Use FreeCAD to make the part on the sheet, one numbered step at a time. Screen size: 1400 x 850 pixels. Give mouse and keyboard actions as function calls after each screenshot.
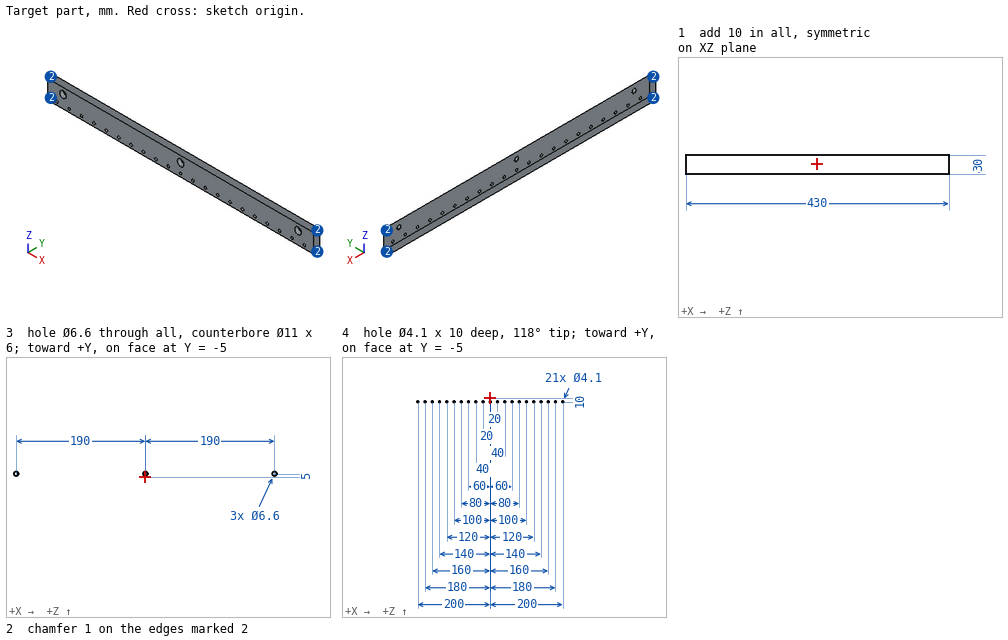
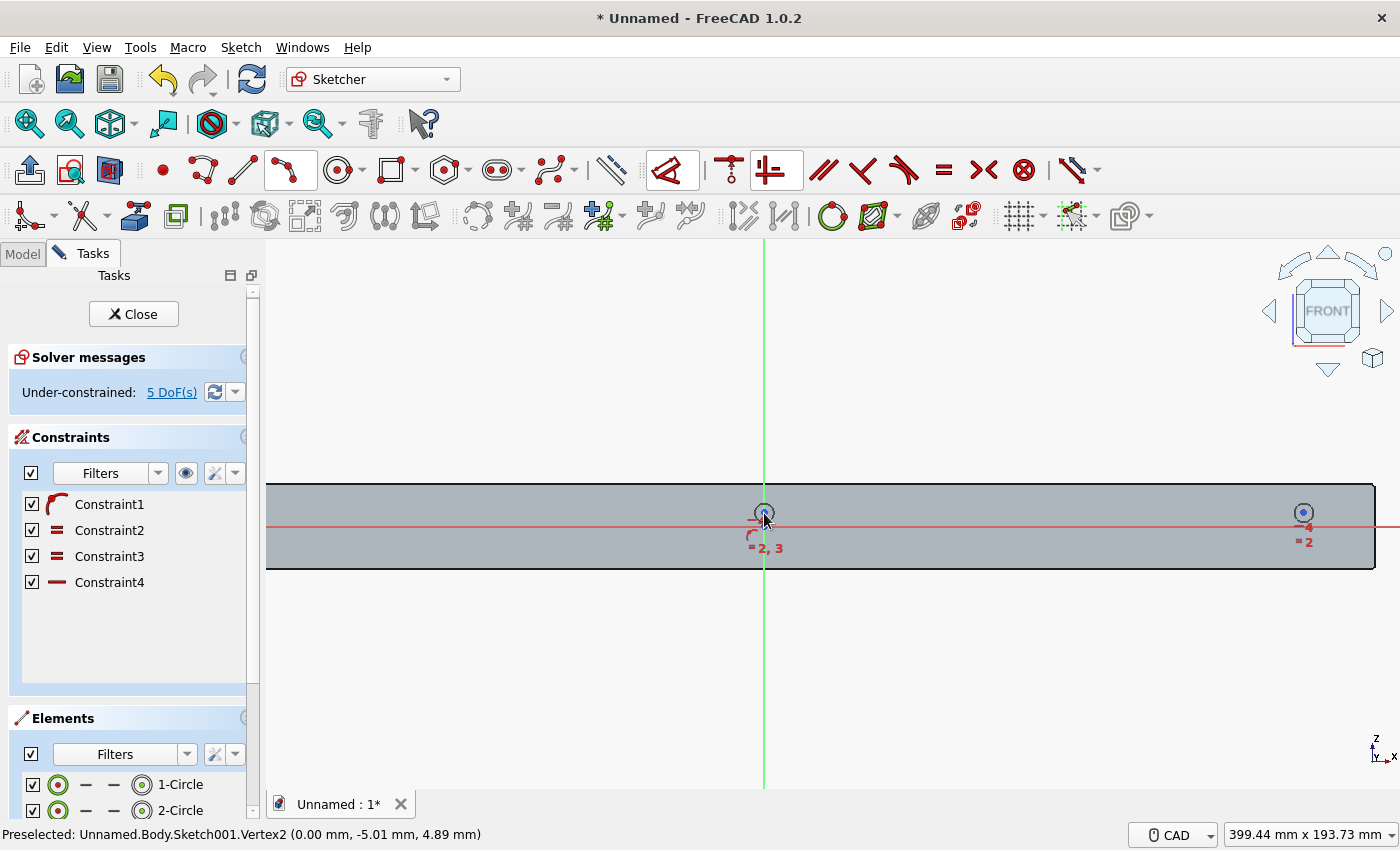
click(762, 511)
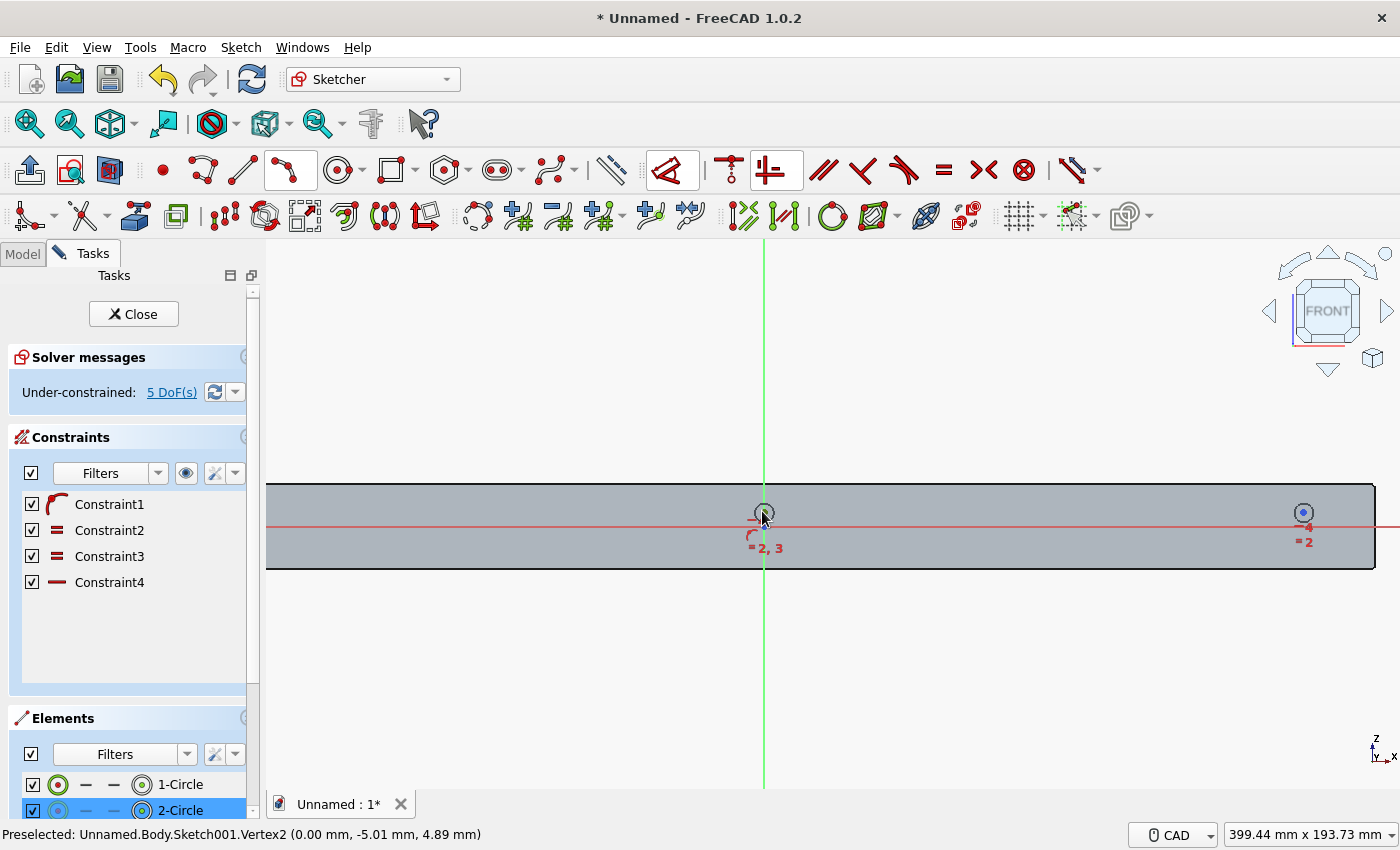
scroll(765, 513, down, 3)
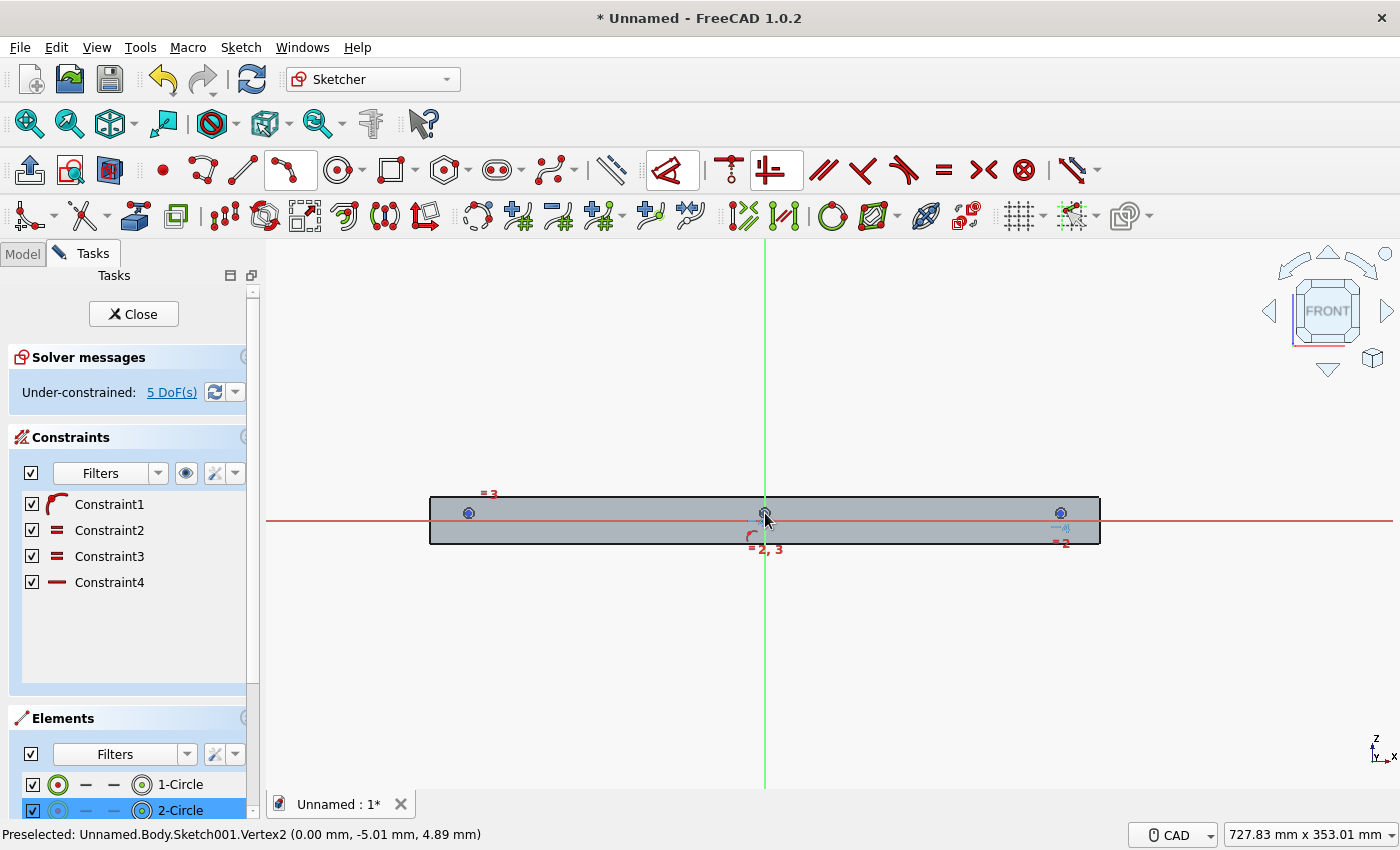
click(469, 513)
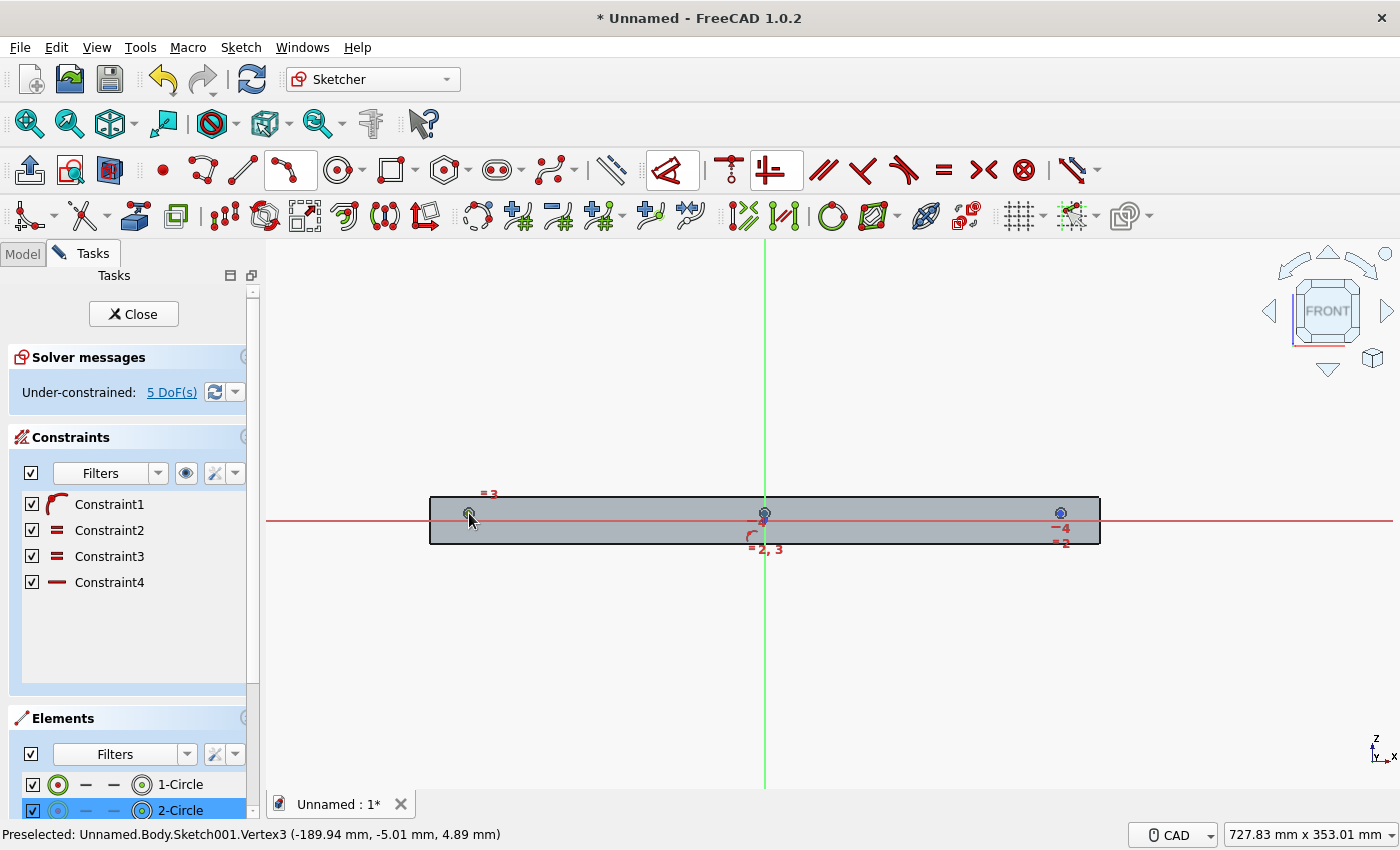
click(798, 170)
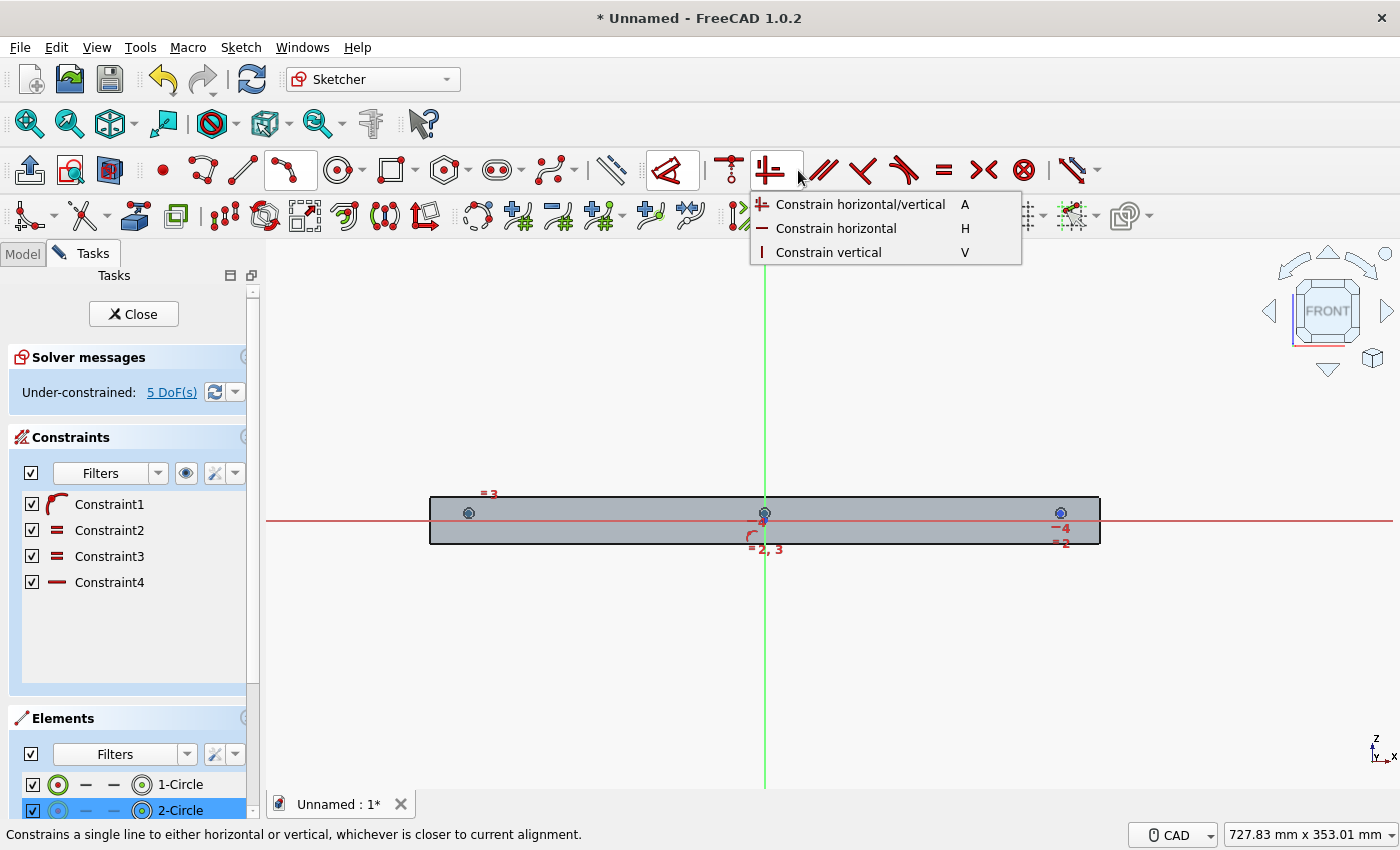
click(886, 228)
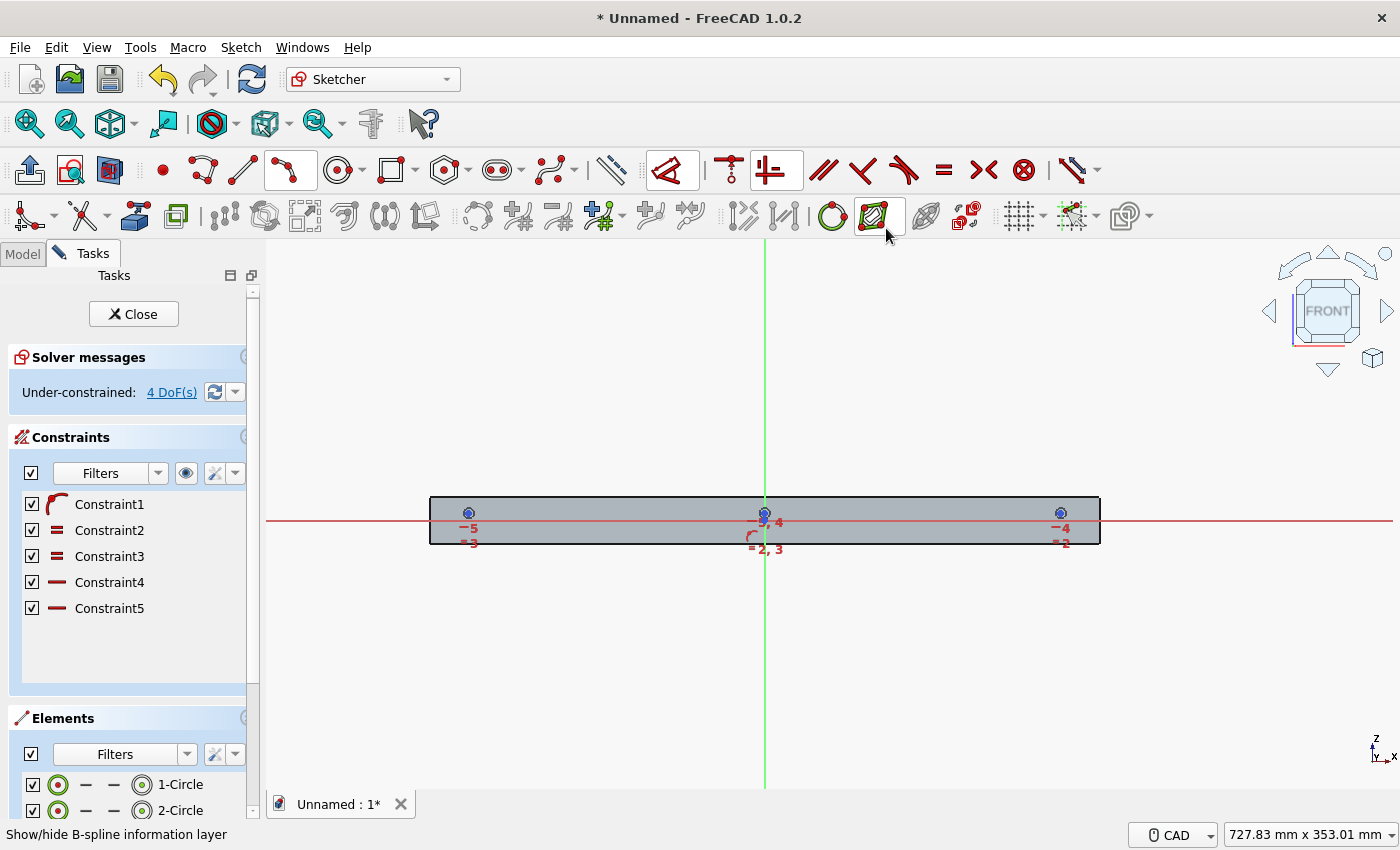
scroll(1065, 517, up, 7)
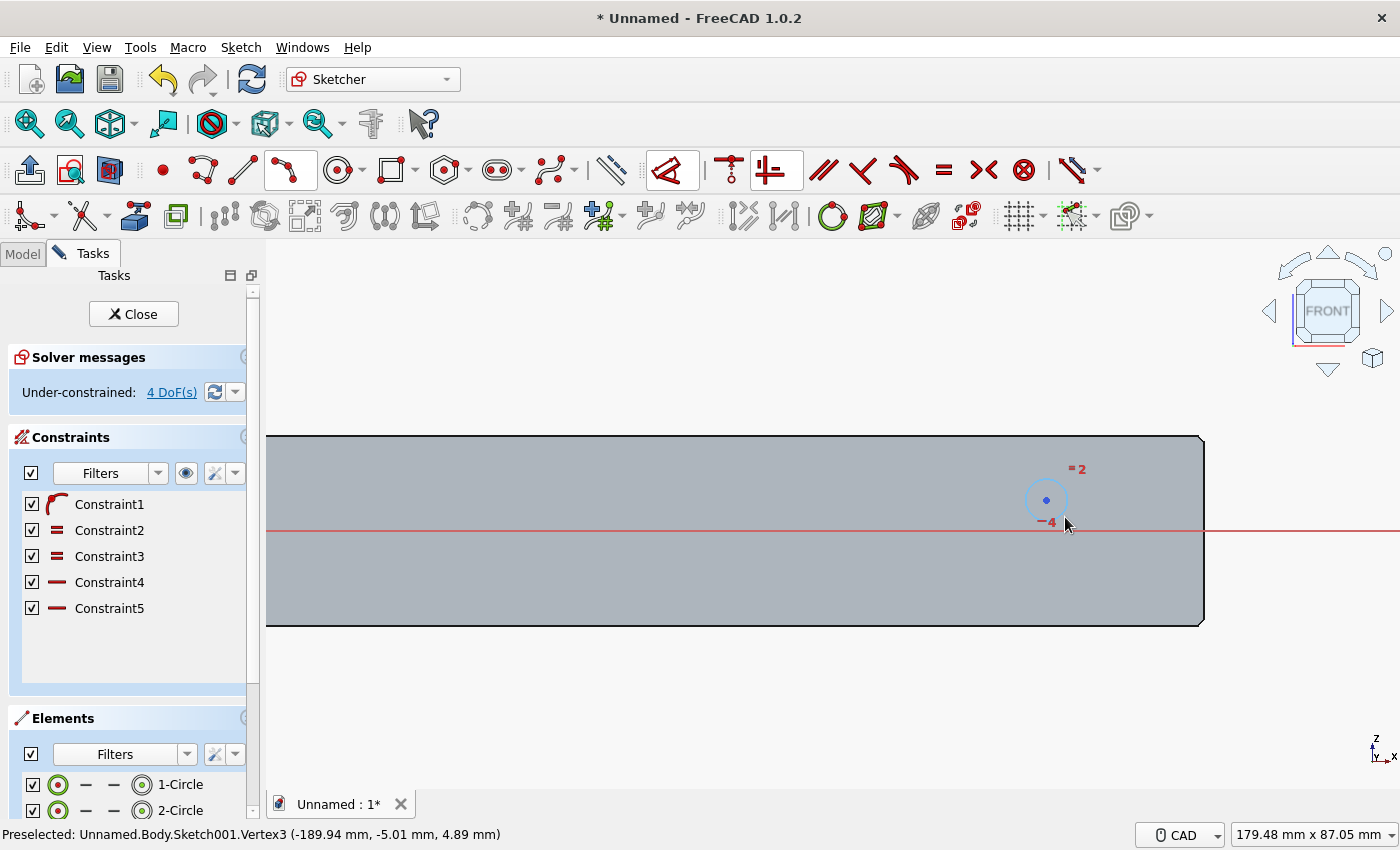
click(1061, 515)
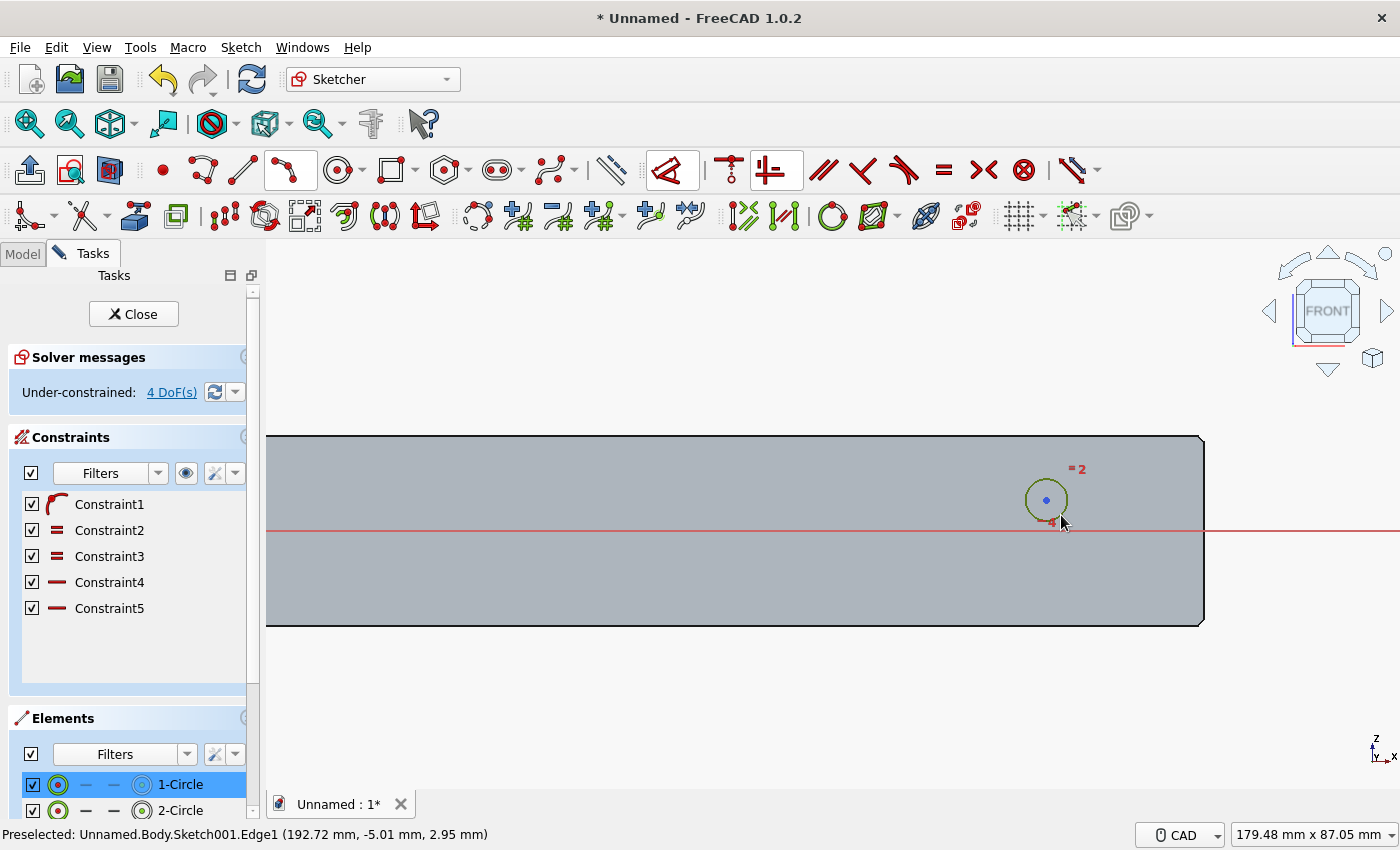
click(694, 170)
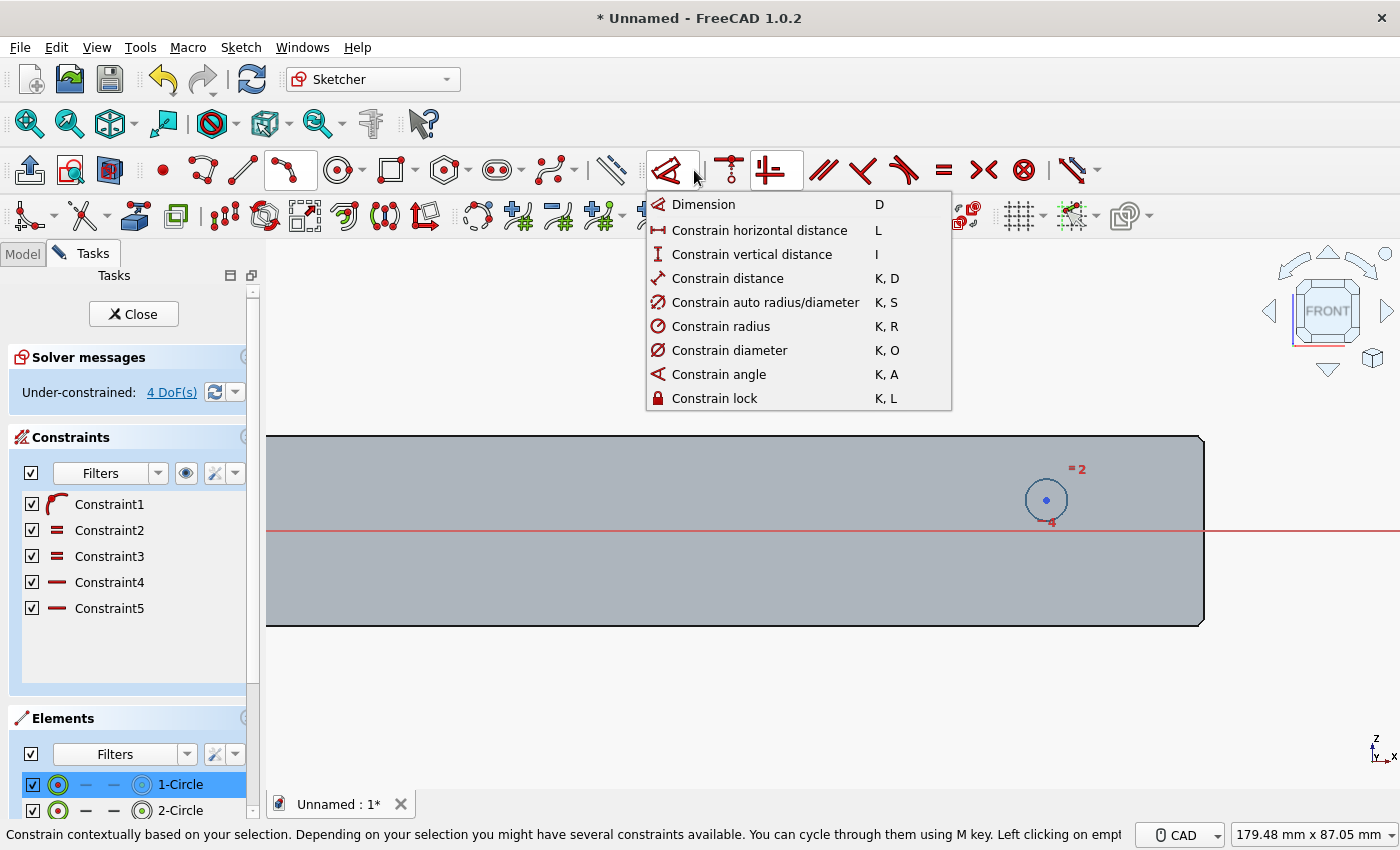
click(799, 350)